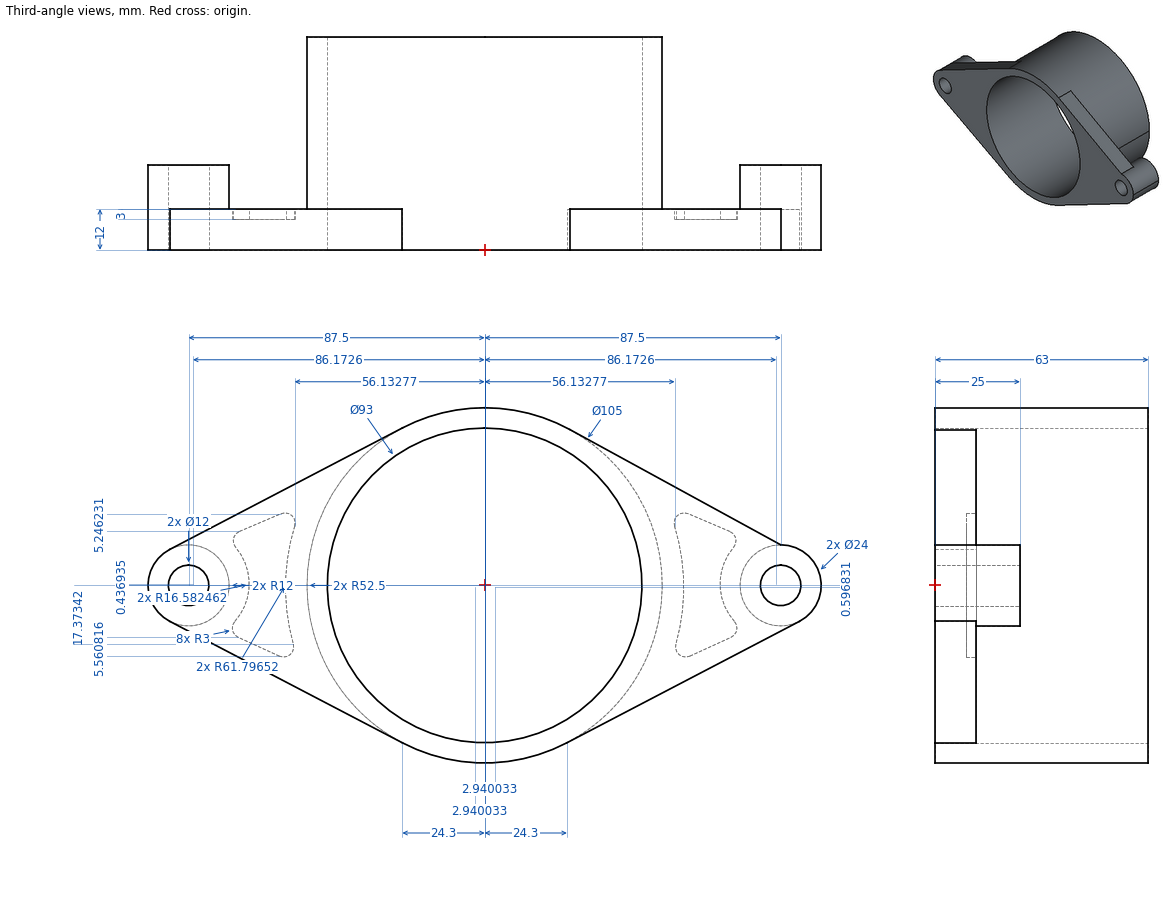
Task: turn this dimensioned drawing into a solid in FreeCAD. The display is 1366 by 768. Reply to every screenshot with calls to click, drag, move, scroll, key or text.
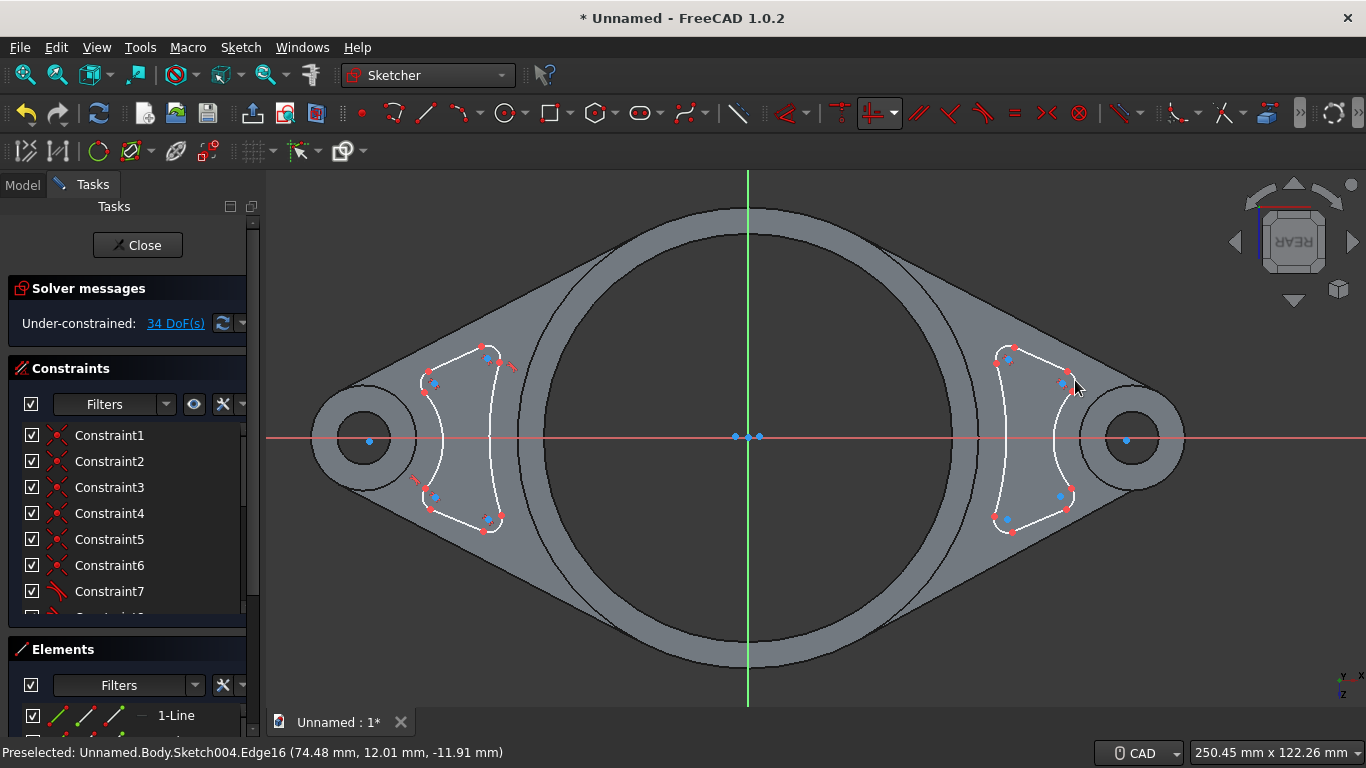
click(1028, 525)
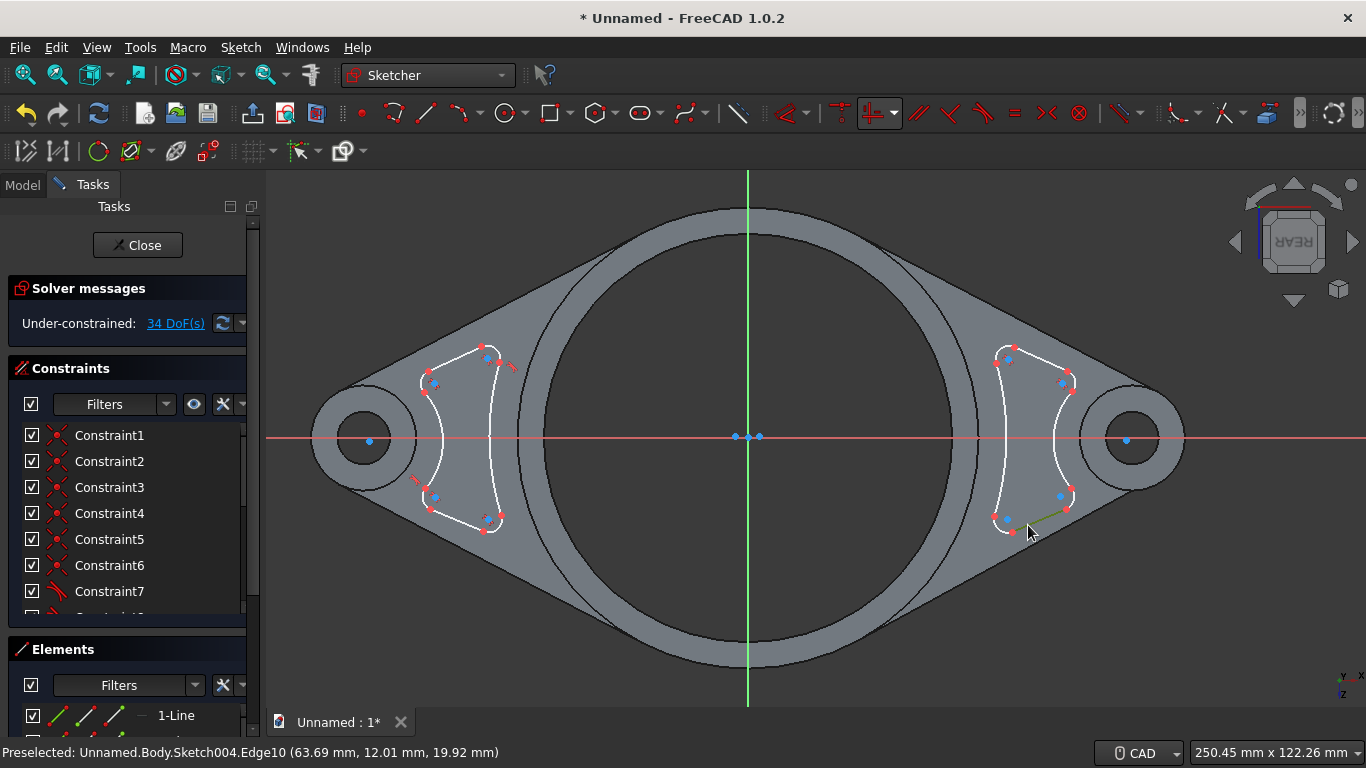
click(999, 529)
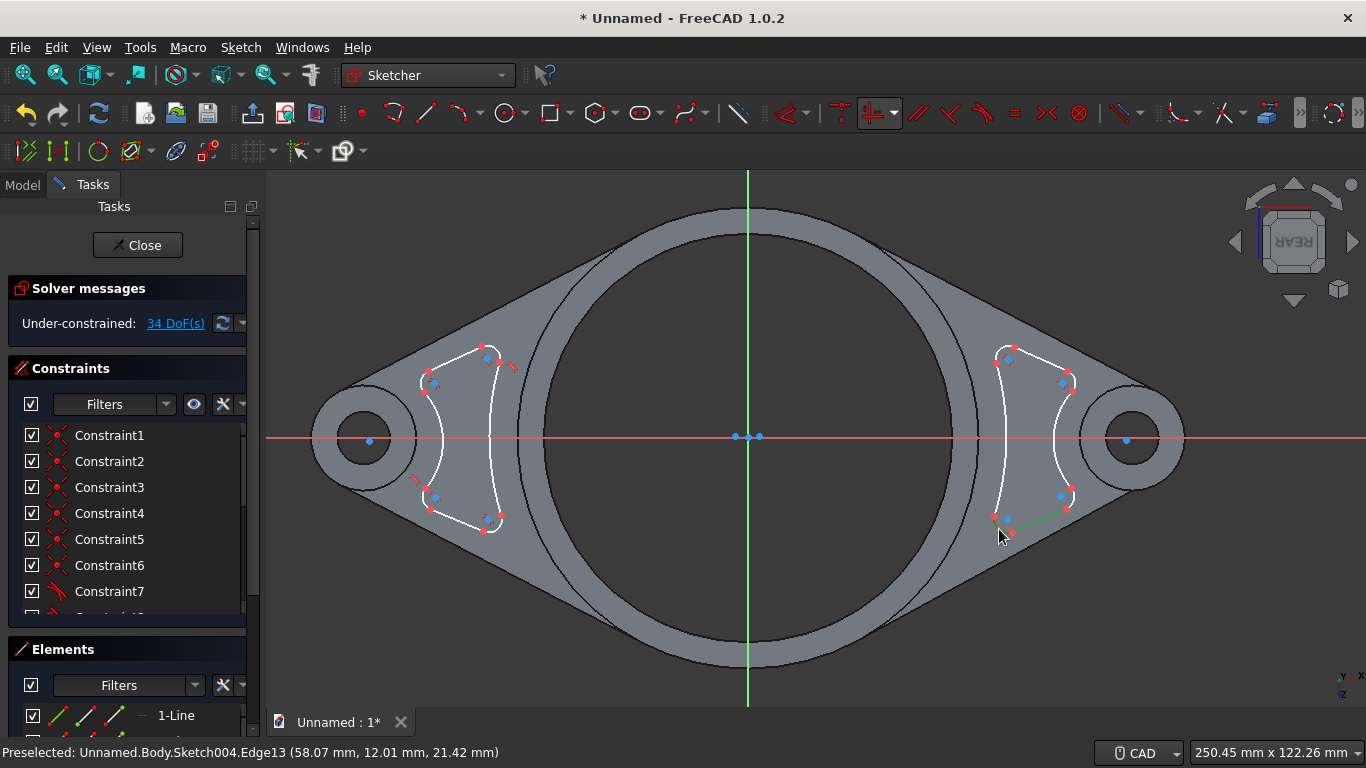
click(984, 114)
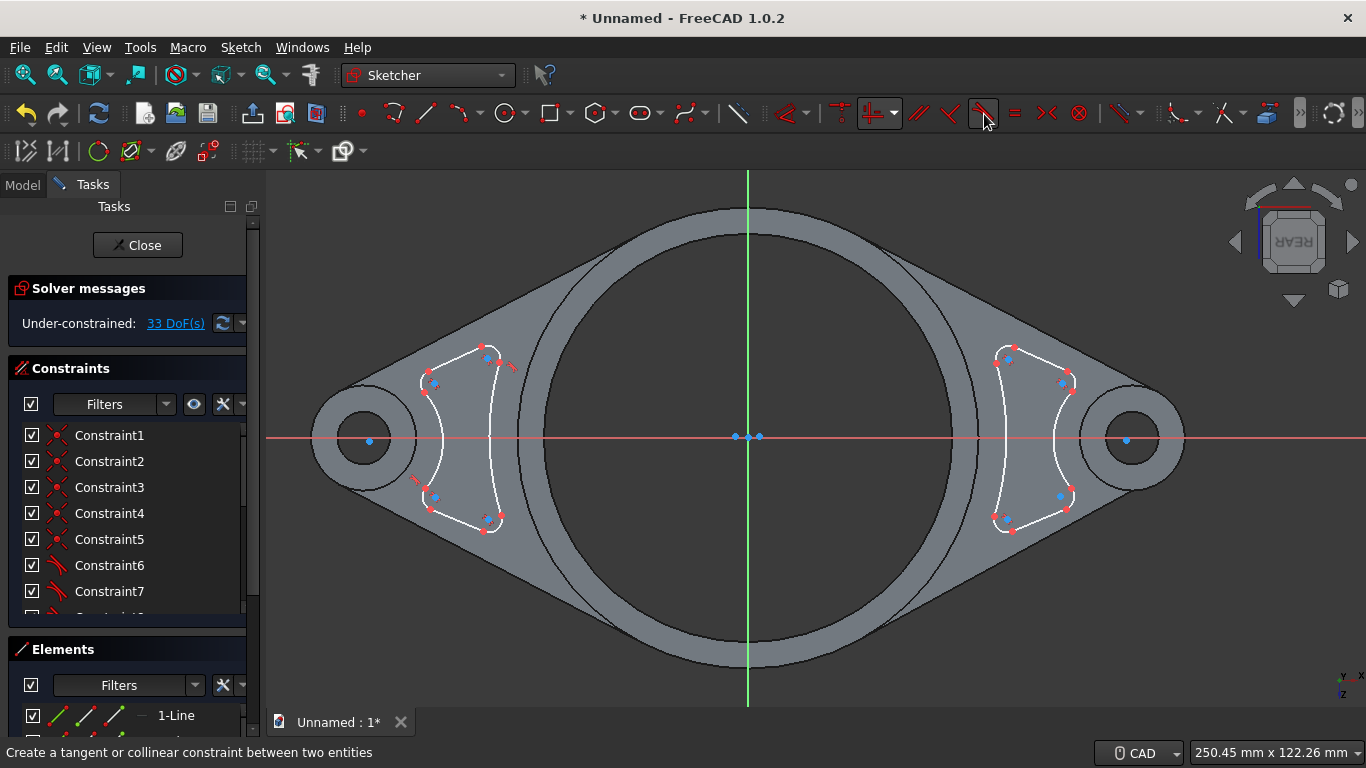
click(1029, 525)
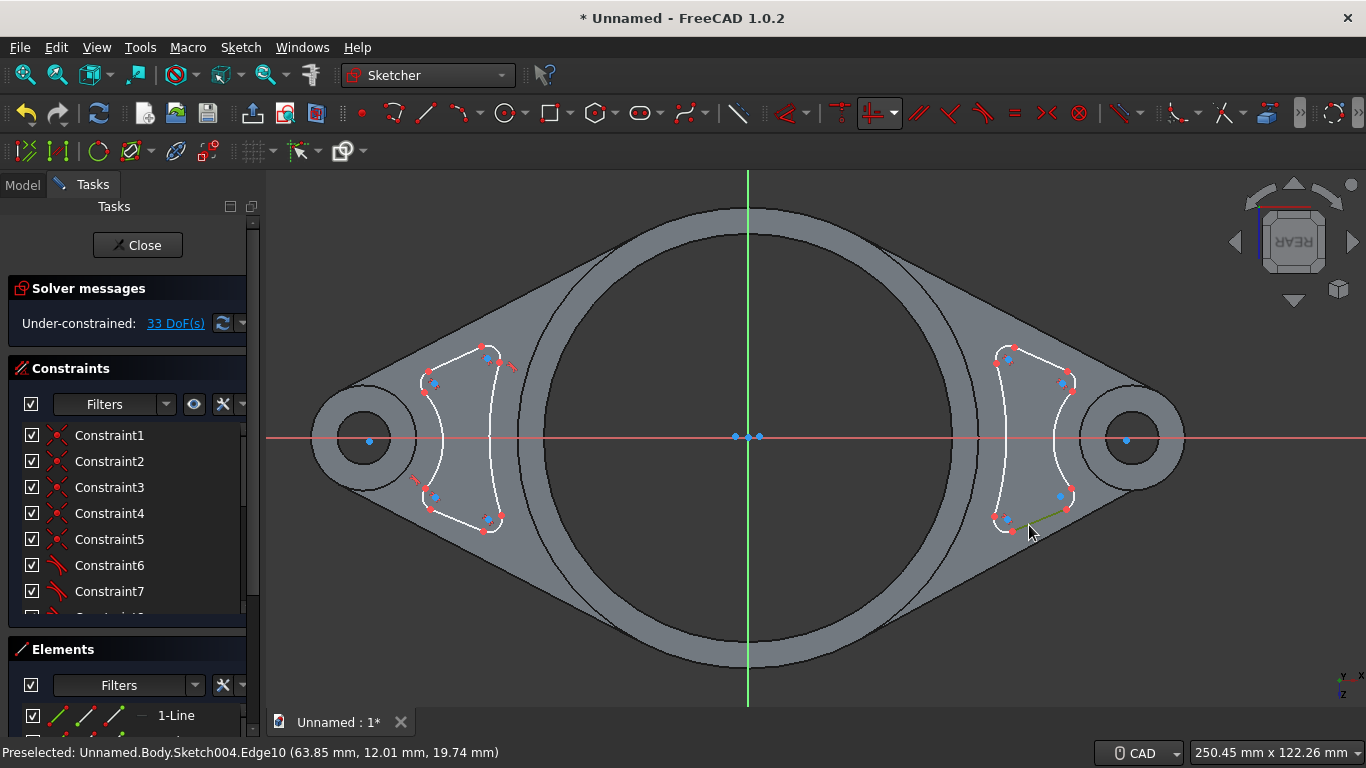
click(1074, 500)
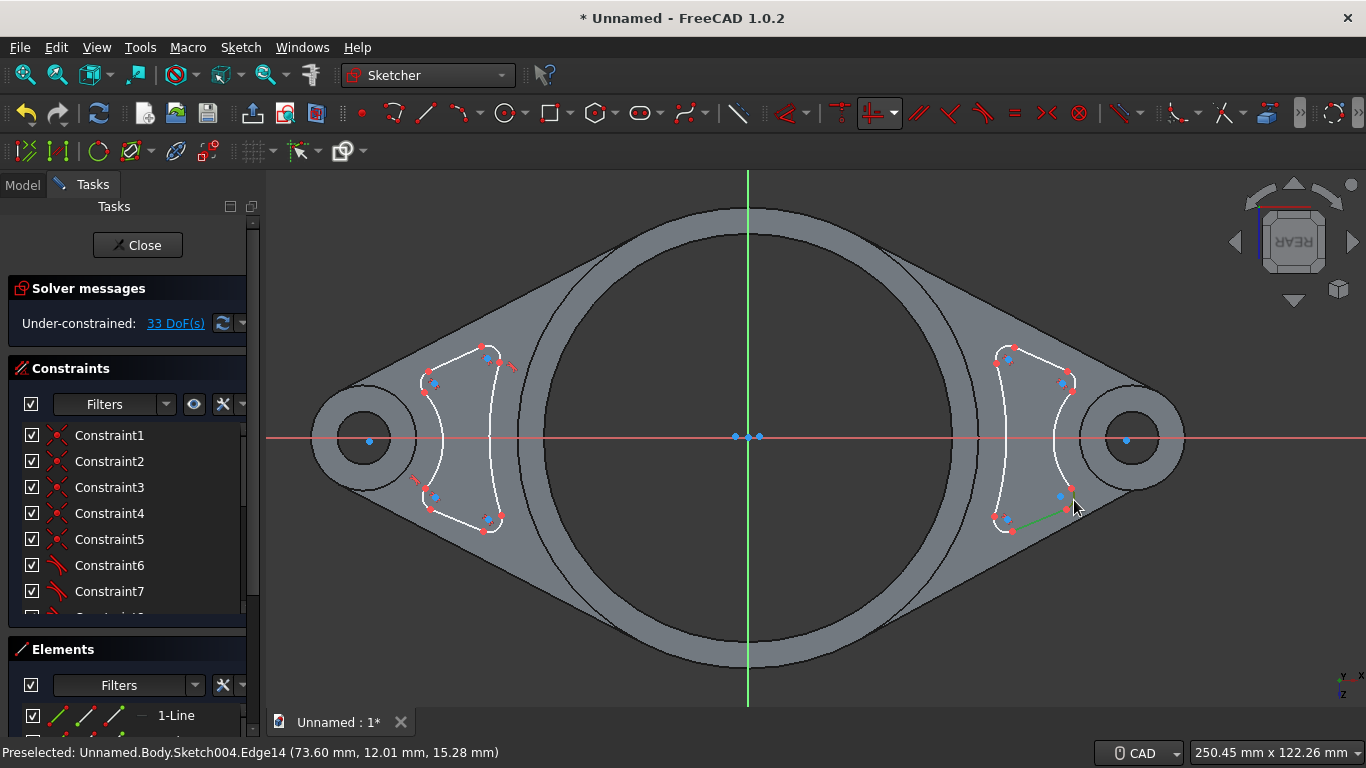
click(984, 114)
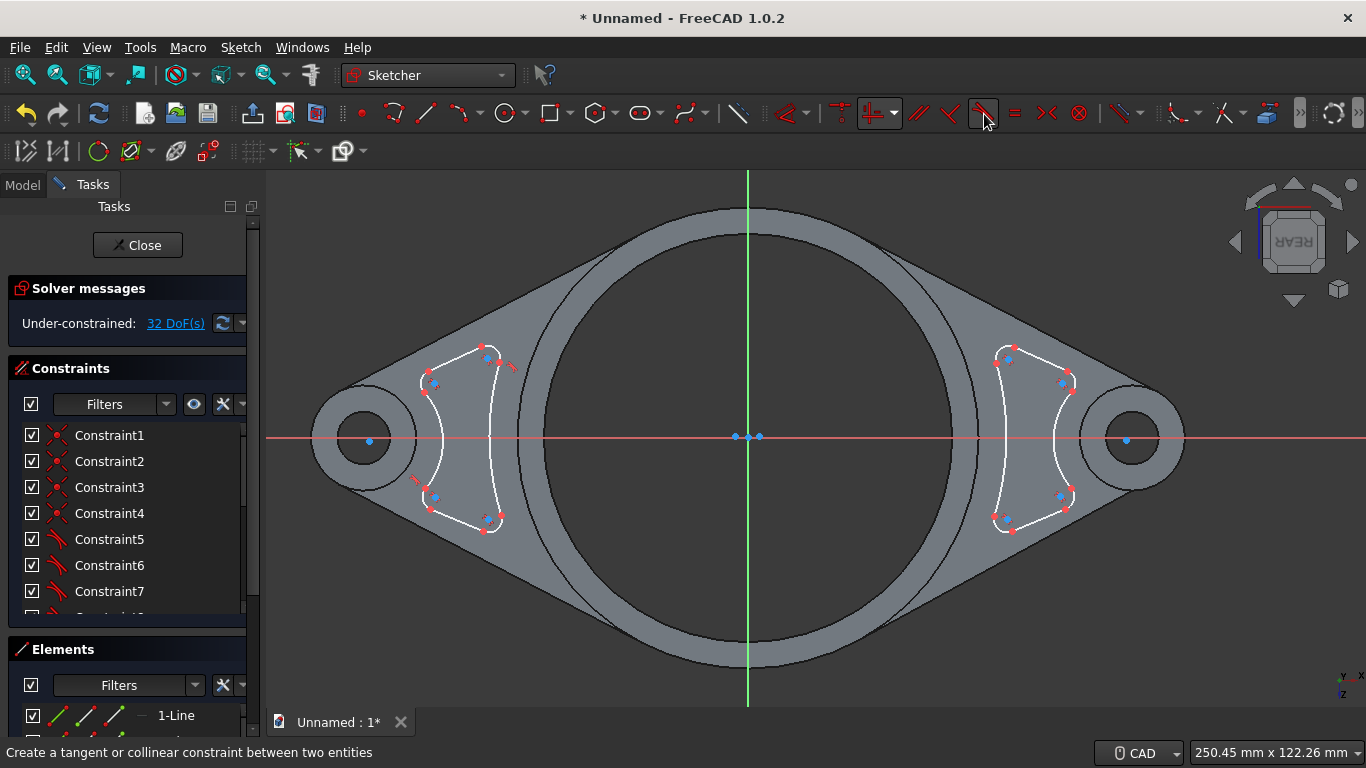
click(1000, 349)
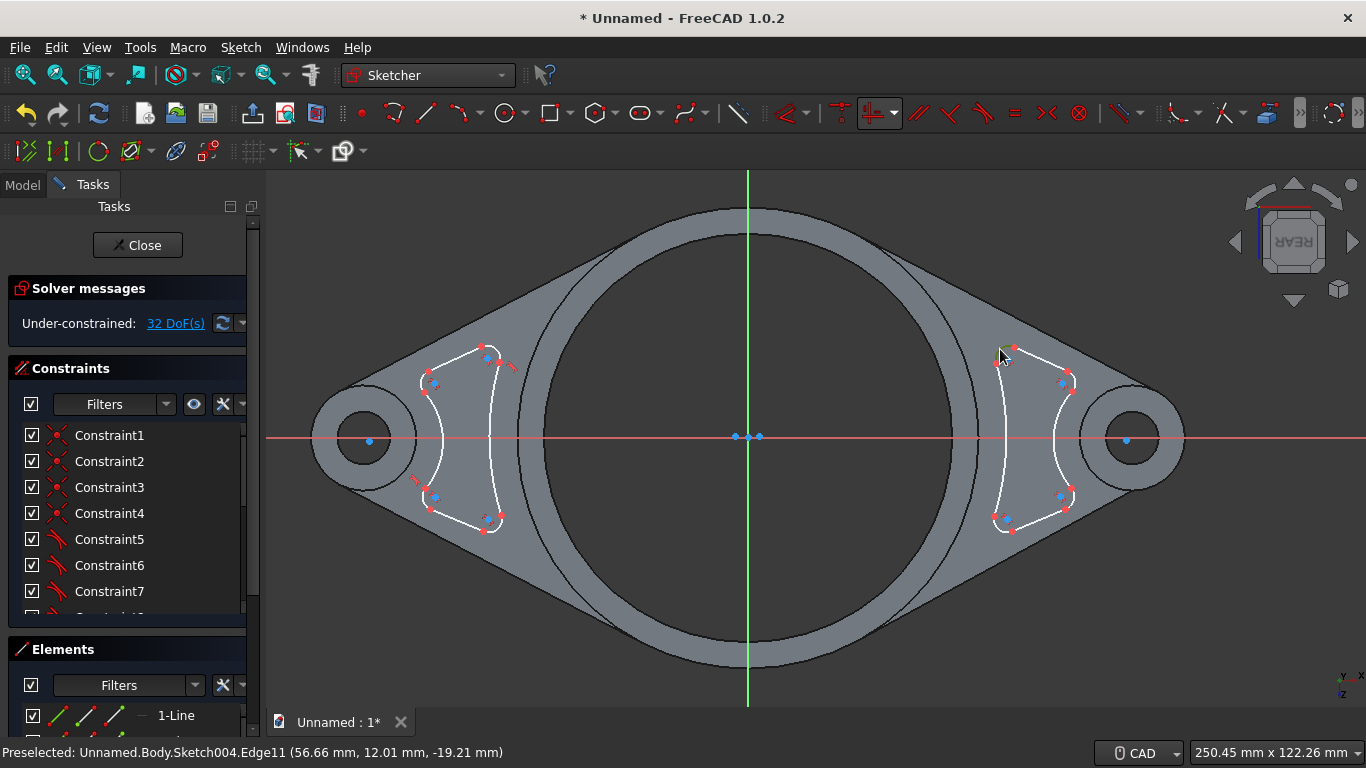
click(1004, 471)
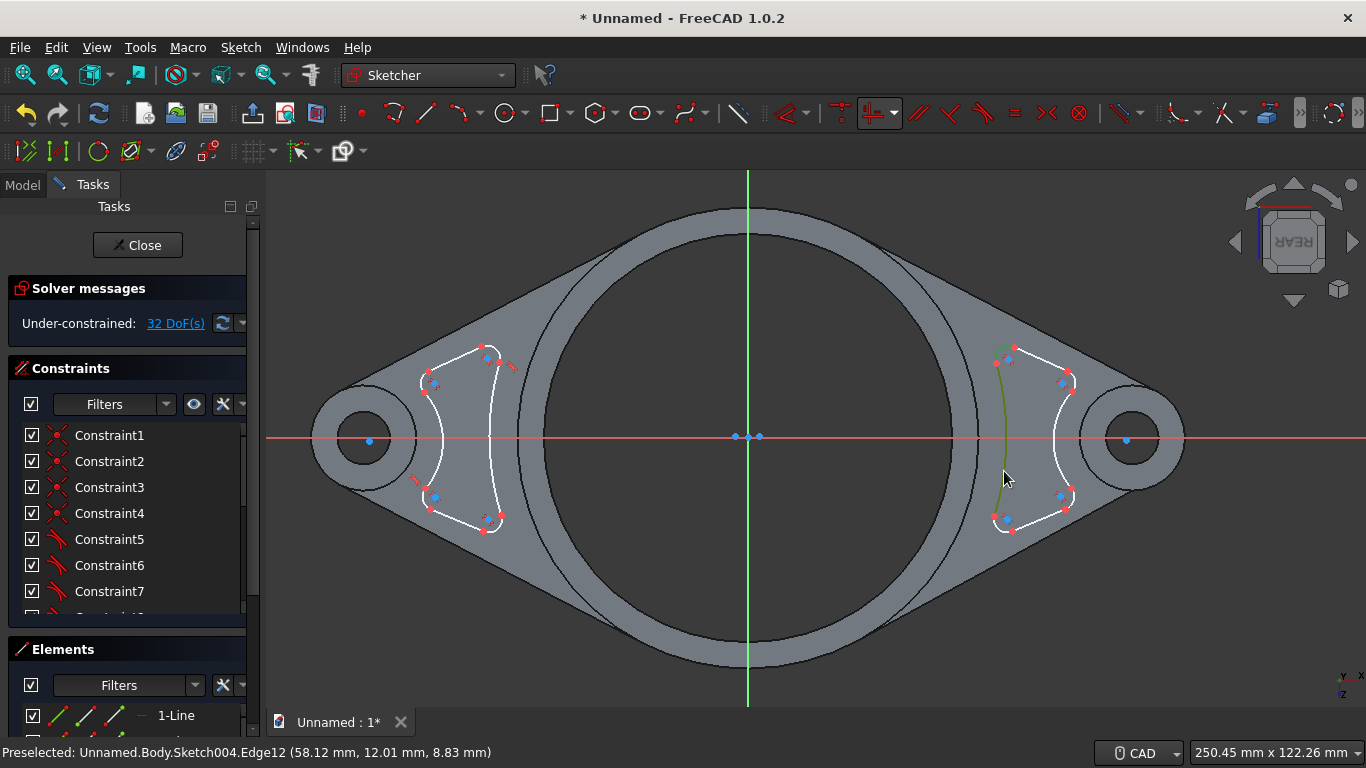
key(t)